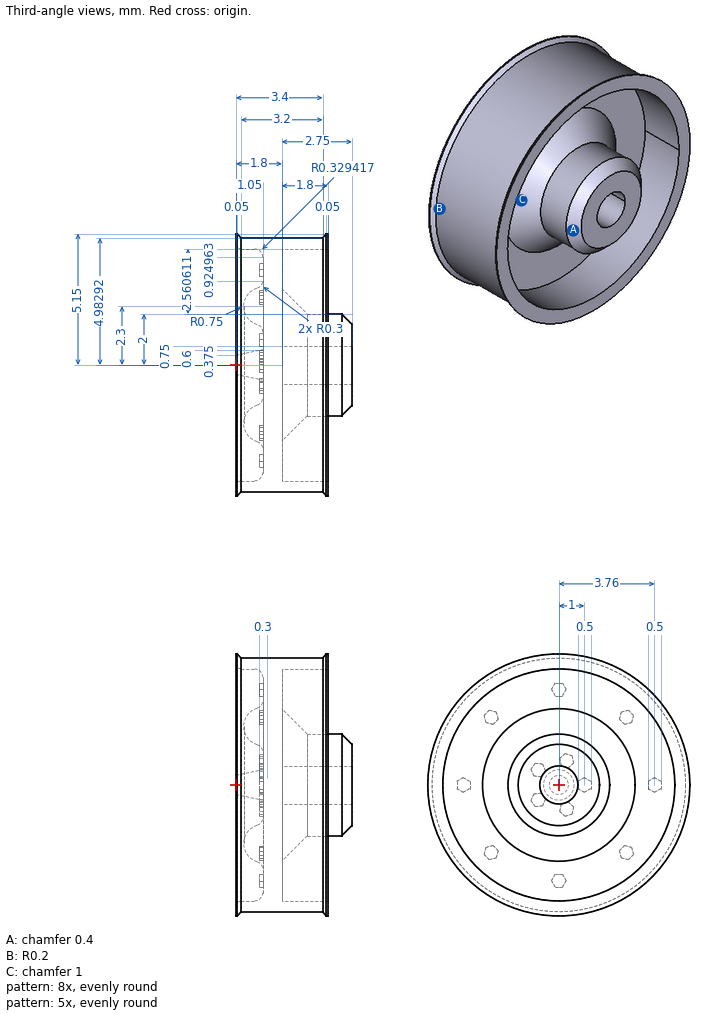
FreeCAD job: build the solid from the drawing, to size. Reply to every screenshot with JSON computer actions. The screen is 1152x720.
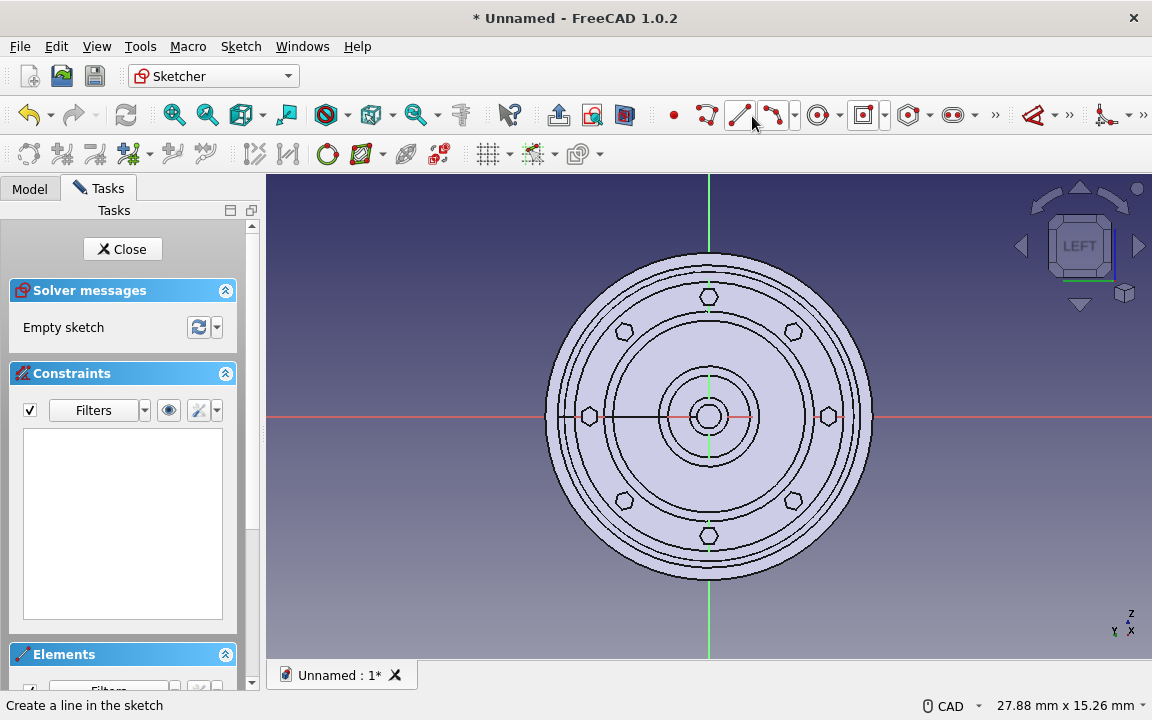
{"action": "left_click", "coordinate": [625, 116]}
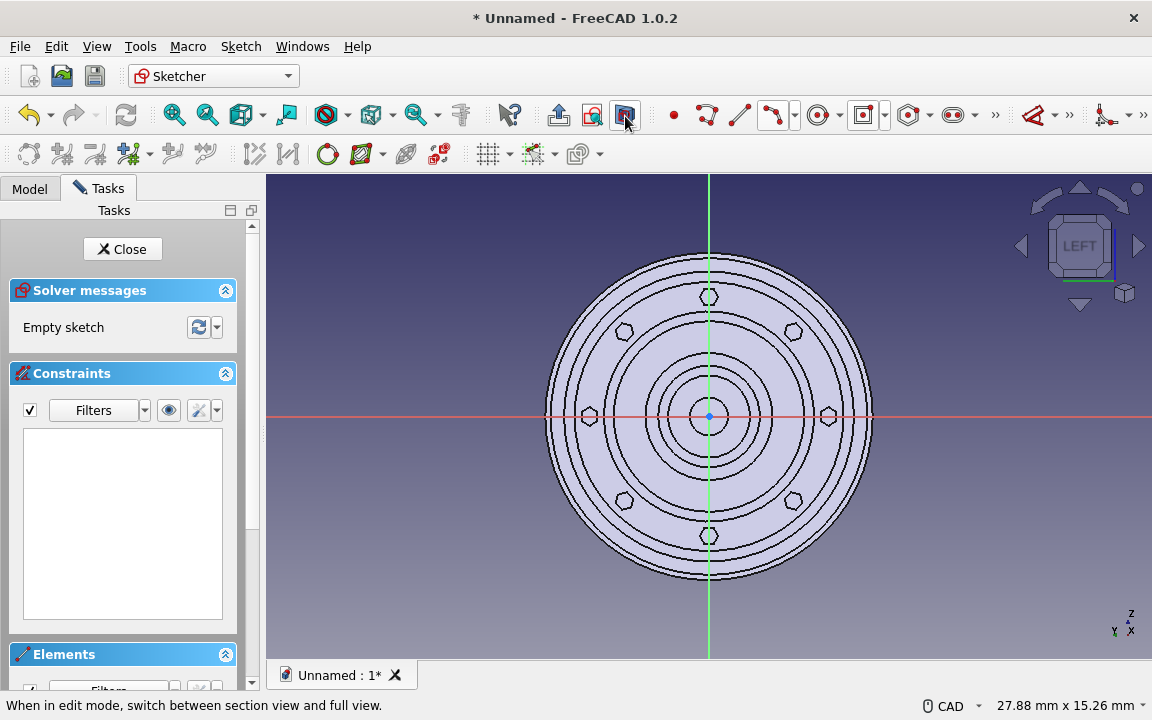
{"action": "scroll", "coordinate": [693, 416], "scroll_direction": "up", "scroll_amount": 13}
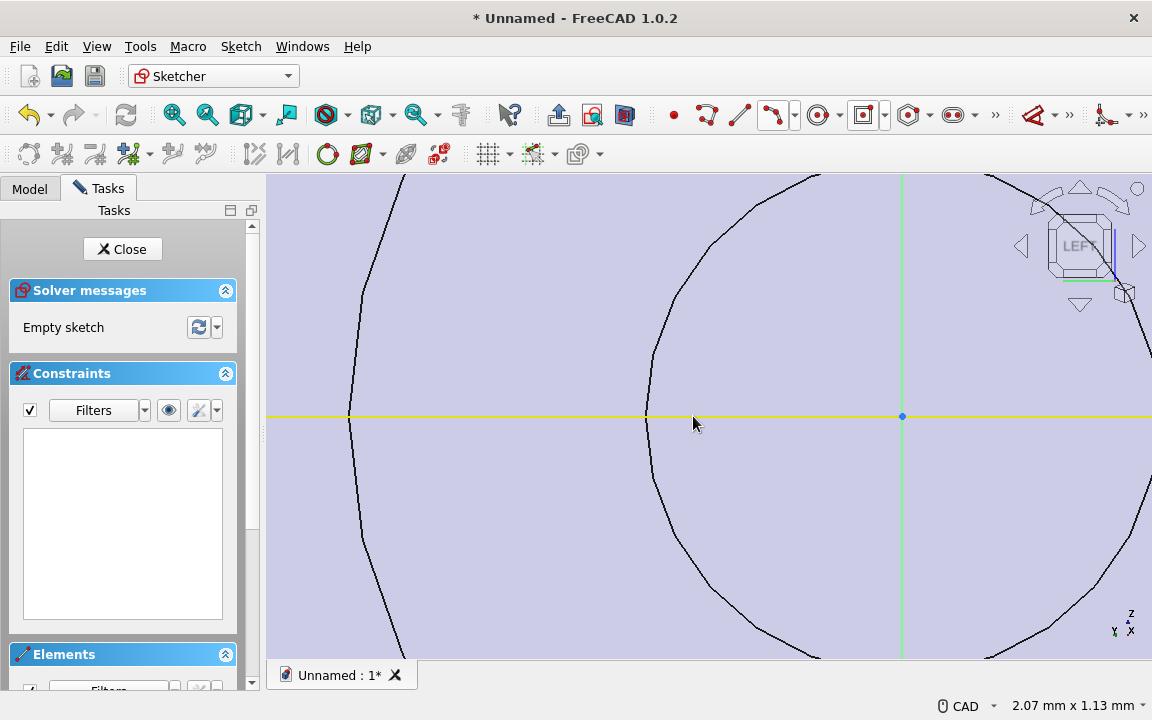
{"action": "left_click", "coordinate": [908, 116]}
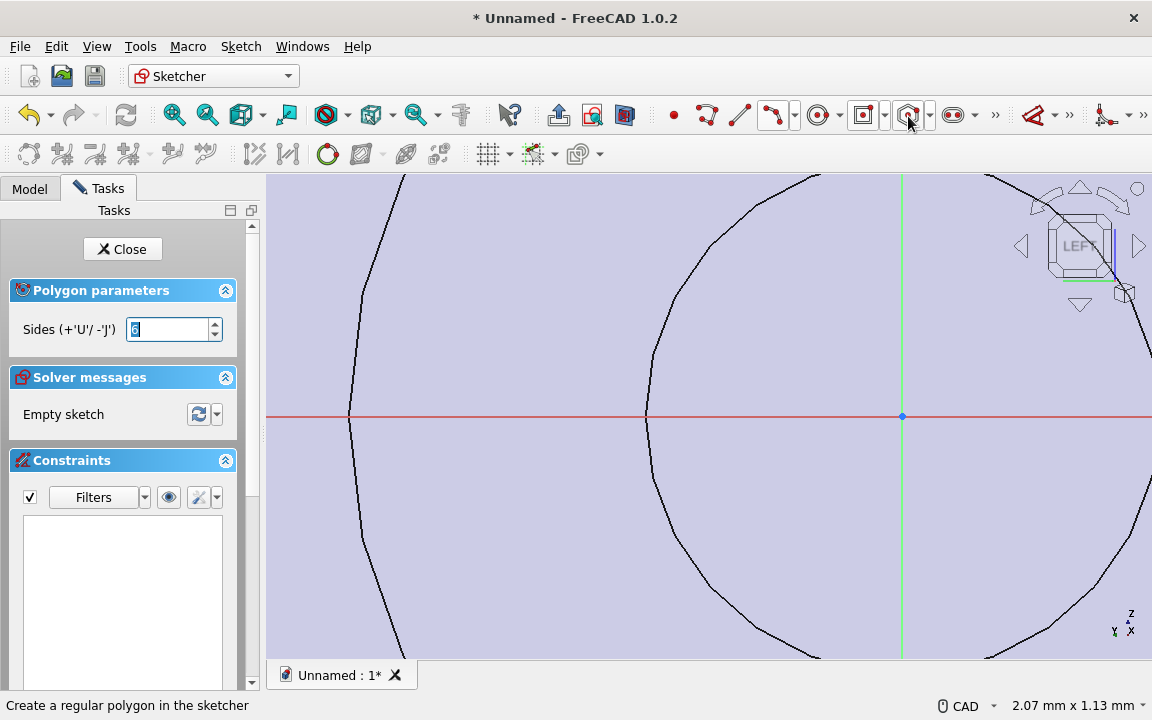
{"action": "left_click", "coordinate": [475, 416]}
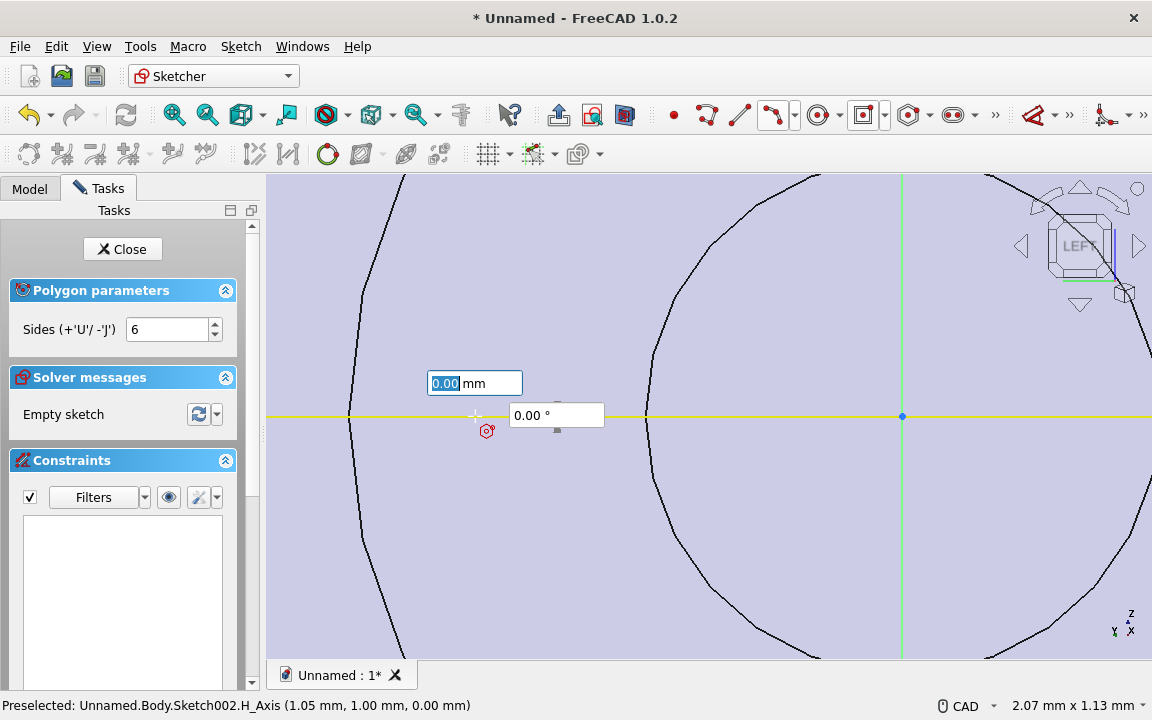
{"action": "left_click", "coordinate": [475, 293]}
{"action": "key", "text": "Escape"}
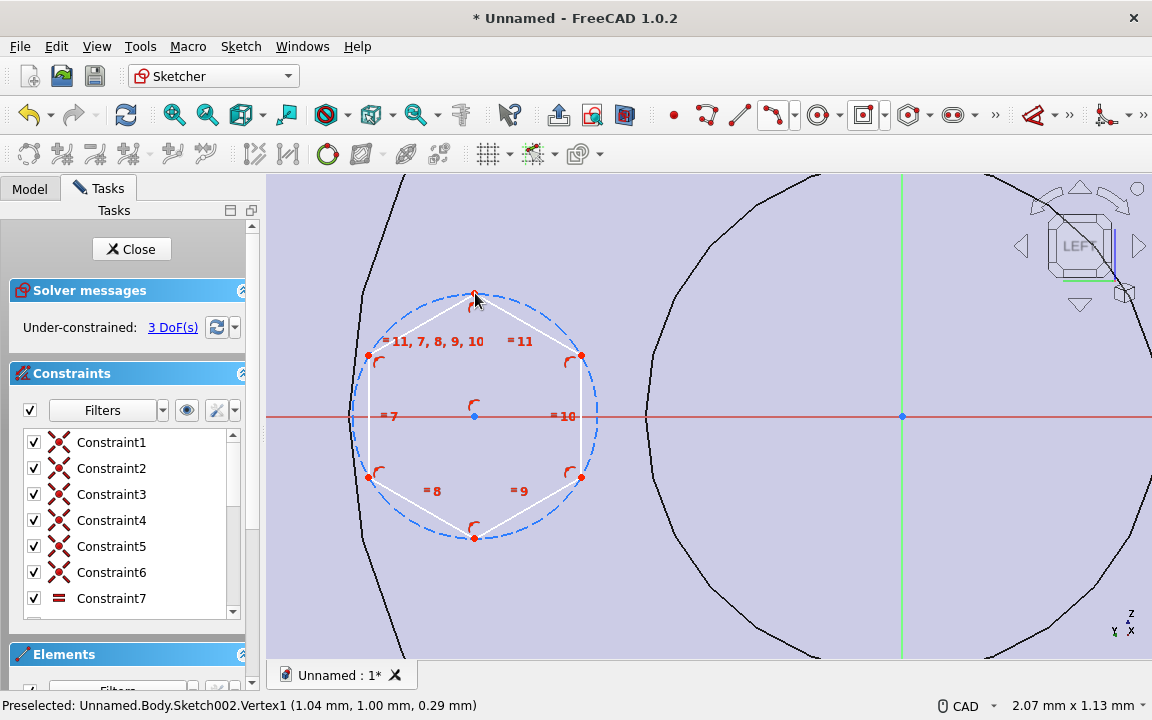
{"action": "left_click", "coordinate": [369, 392]}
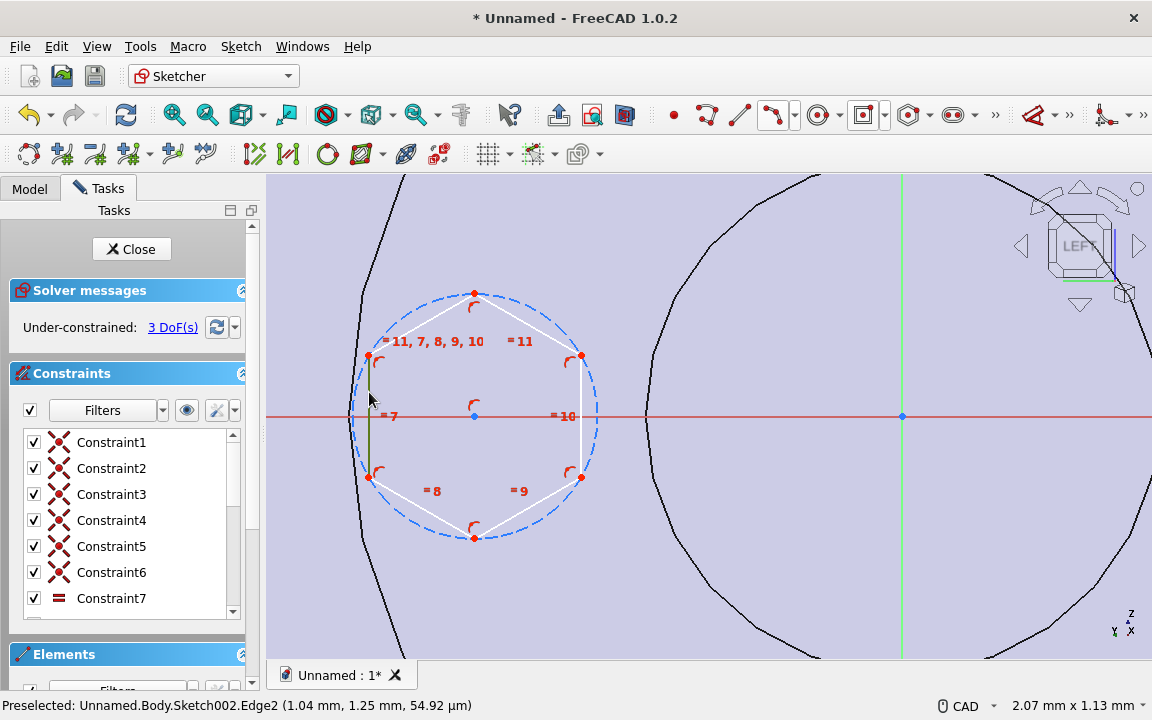
{"action": "key", "text": "v"}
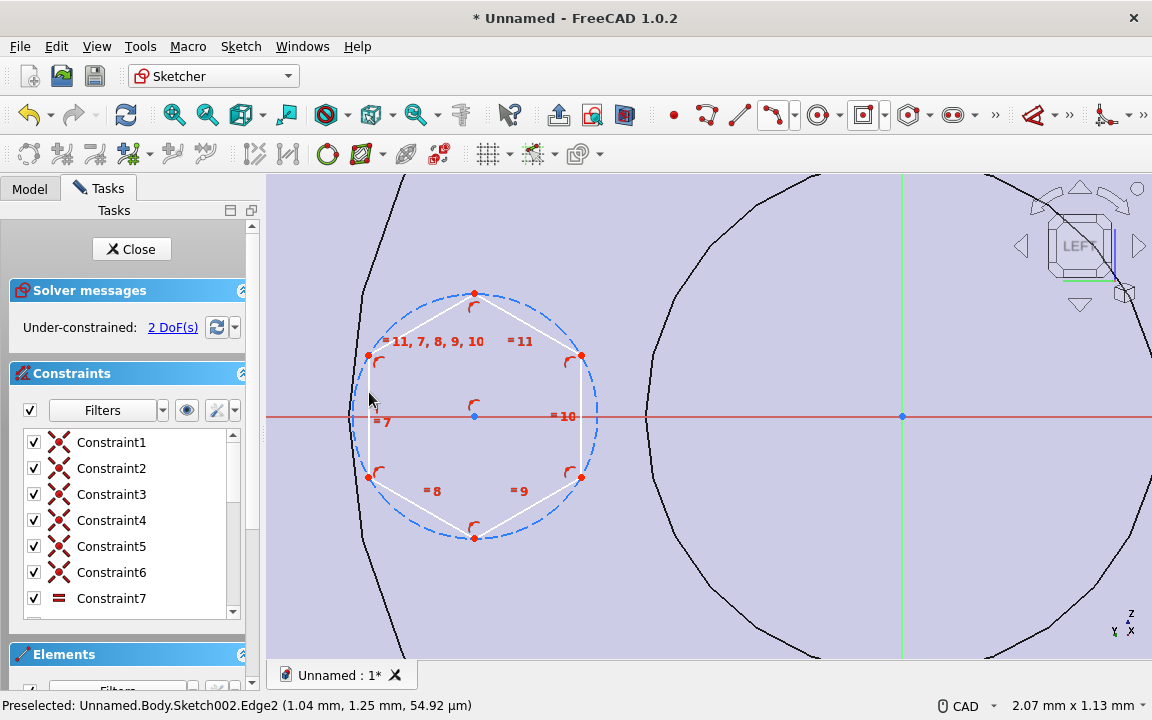
{"action": "left_click", "coordinate": [1032, 116]}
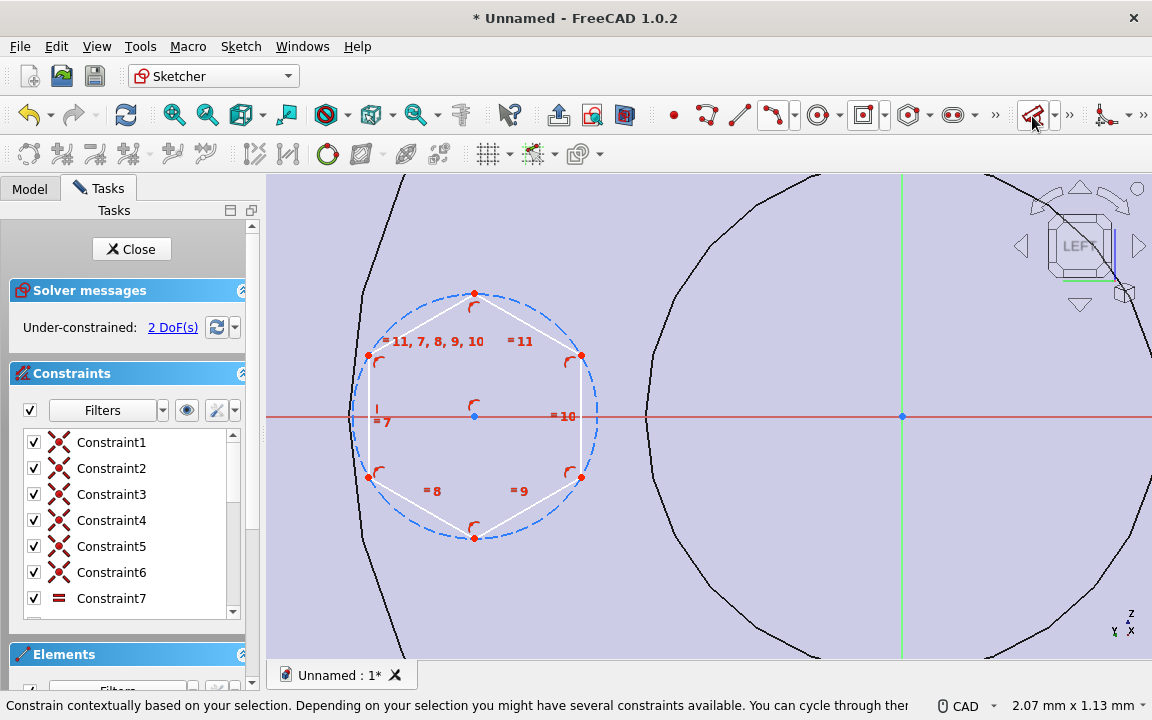
{"action": "left_click", "coordinate": [475, 416]}
{"action": "left_click", "coordinate": [689, 450]}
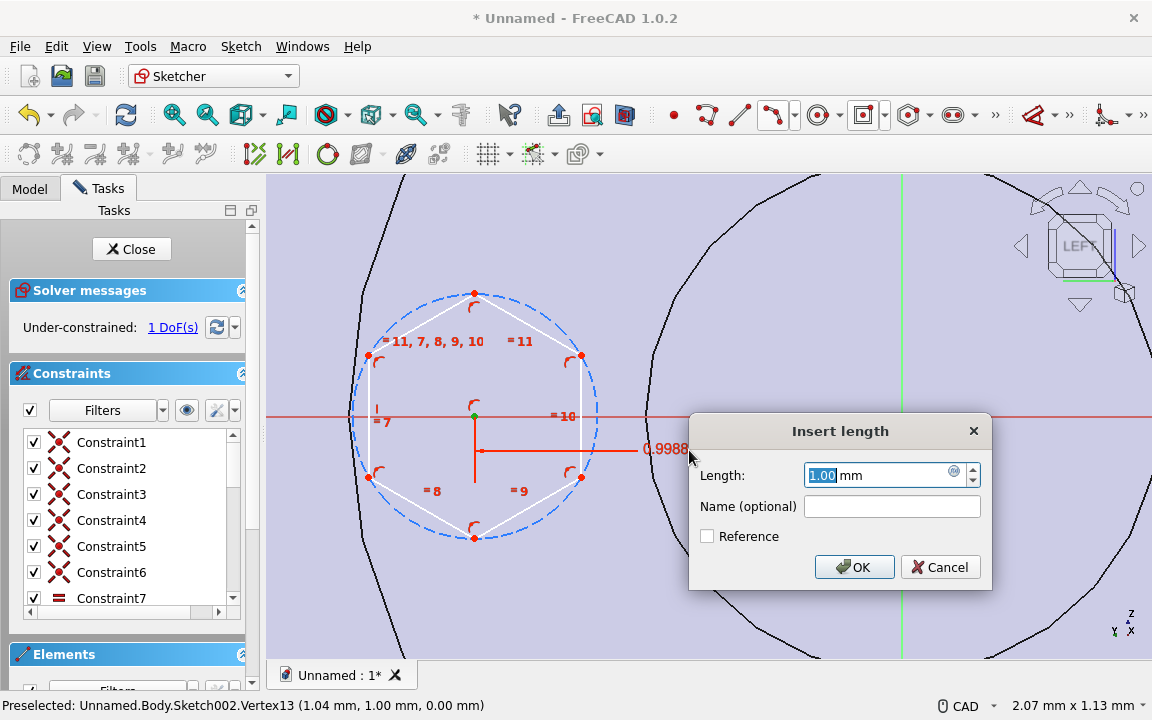
{"action": "type", "text": "1"}
{"action": "key", "text": "Return"}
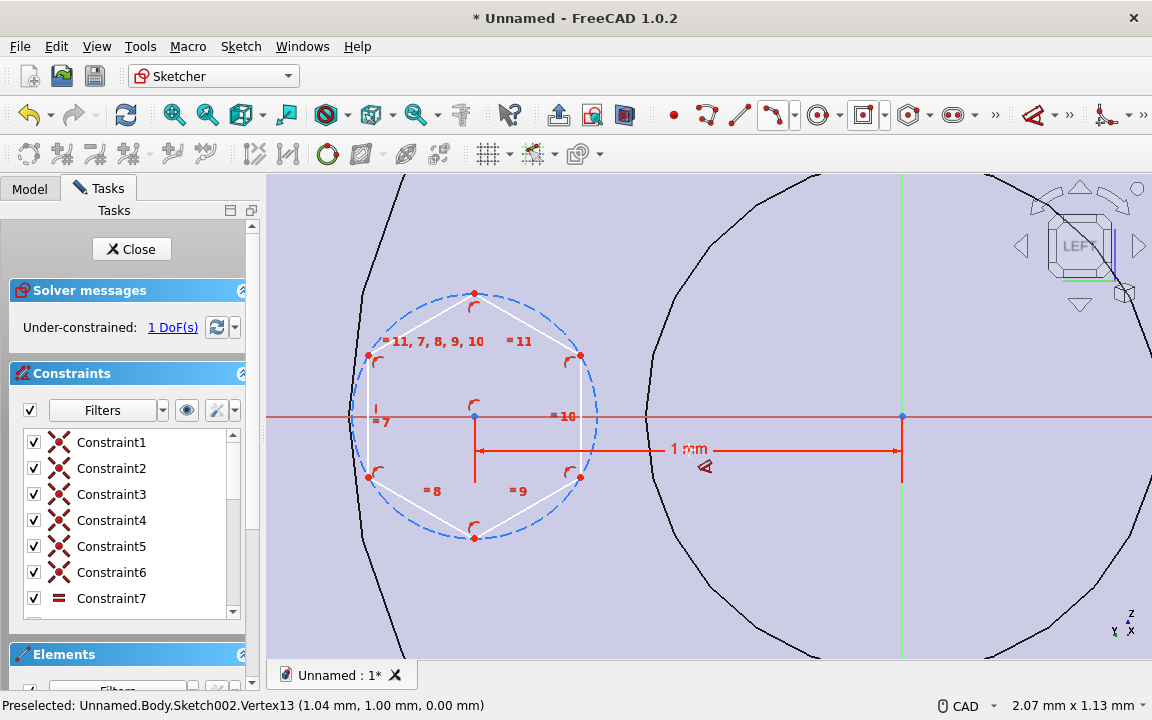
{"action": "left_click", "coordinate": [368, 355]}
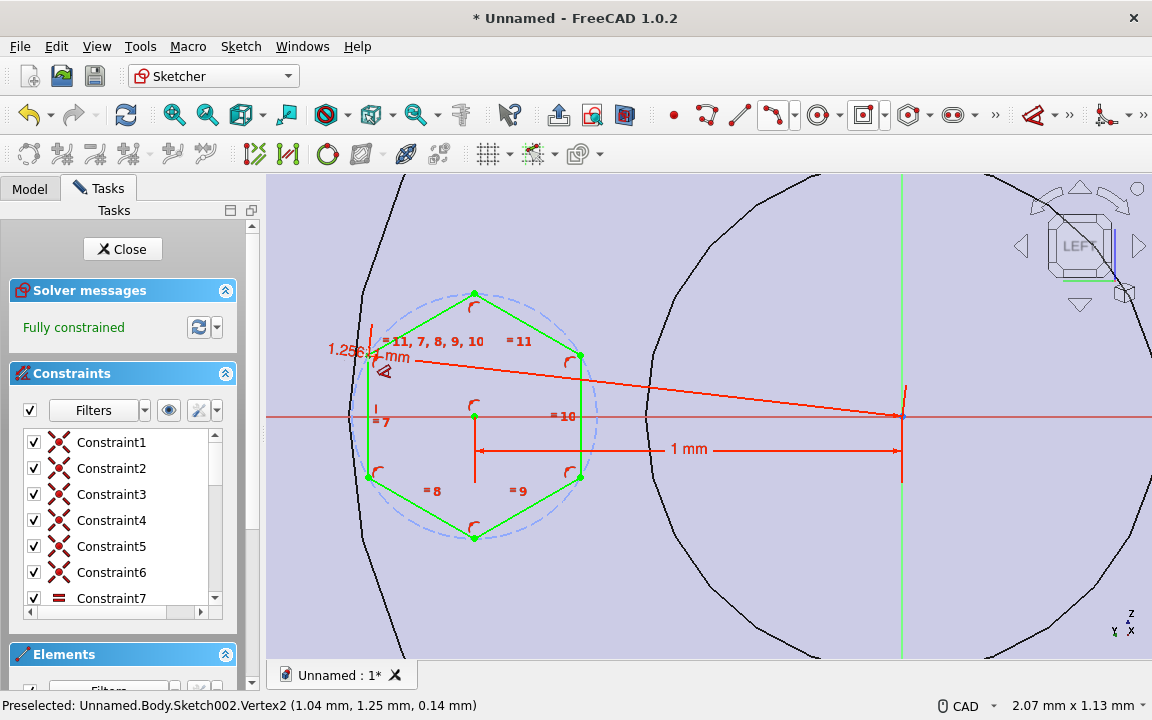
{"action": "left_click", "coordinate": [581, 478]}
{"action": "left_click", "coordinate": [475, 512]}